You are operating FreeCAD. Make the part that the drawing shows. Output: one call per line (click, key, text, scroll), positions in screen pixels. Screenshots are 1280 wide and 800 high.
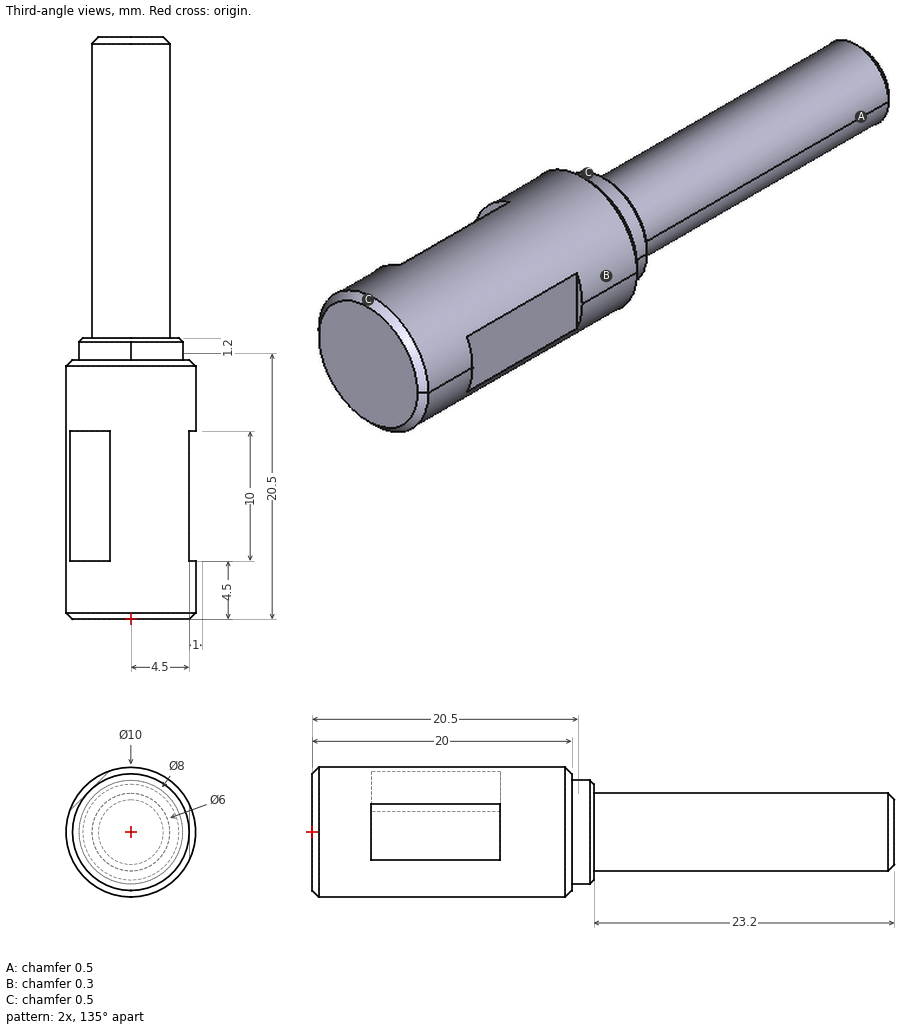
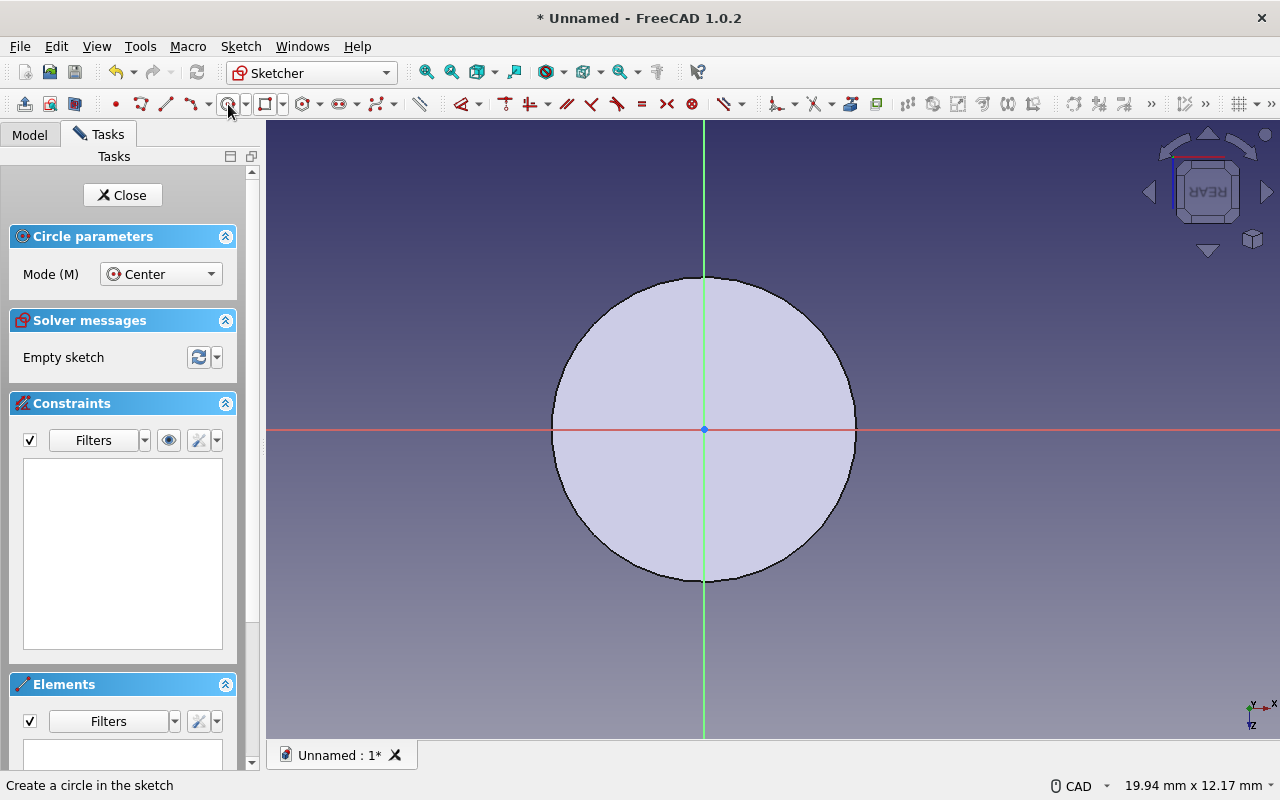
click(704, 429)
move(848, 286)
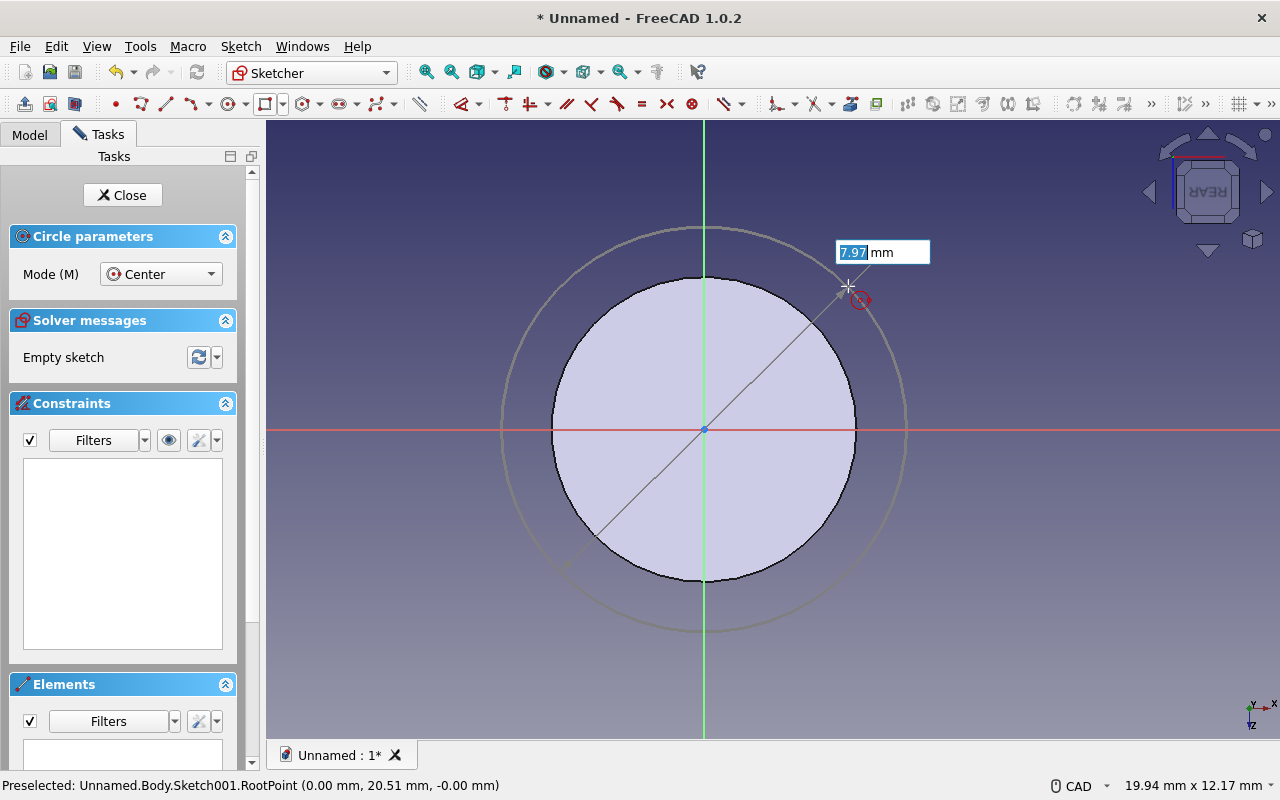
text(8)
key(Return)
key(Escape)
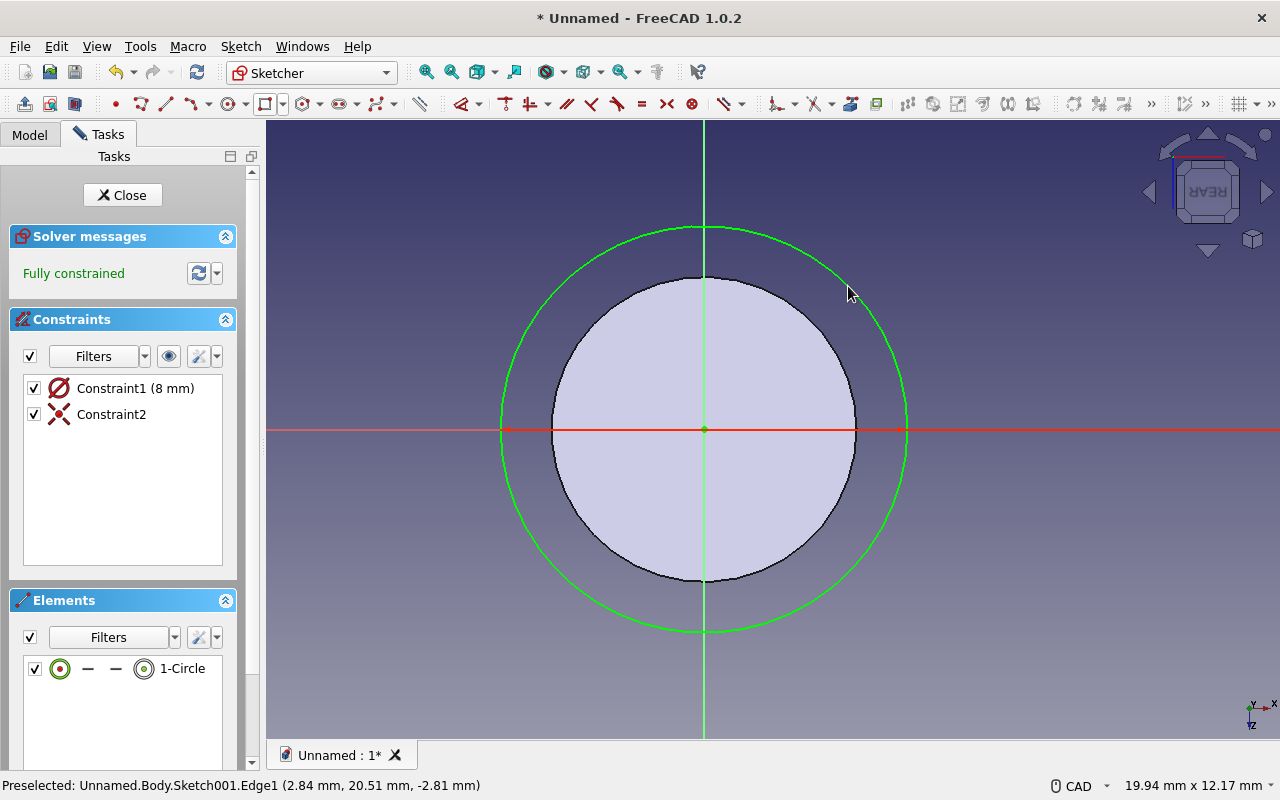
click(123, 195)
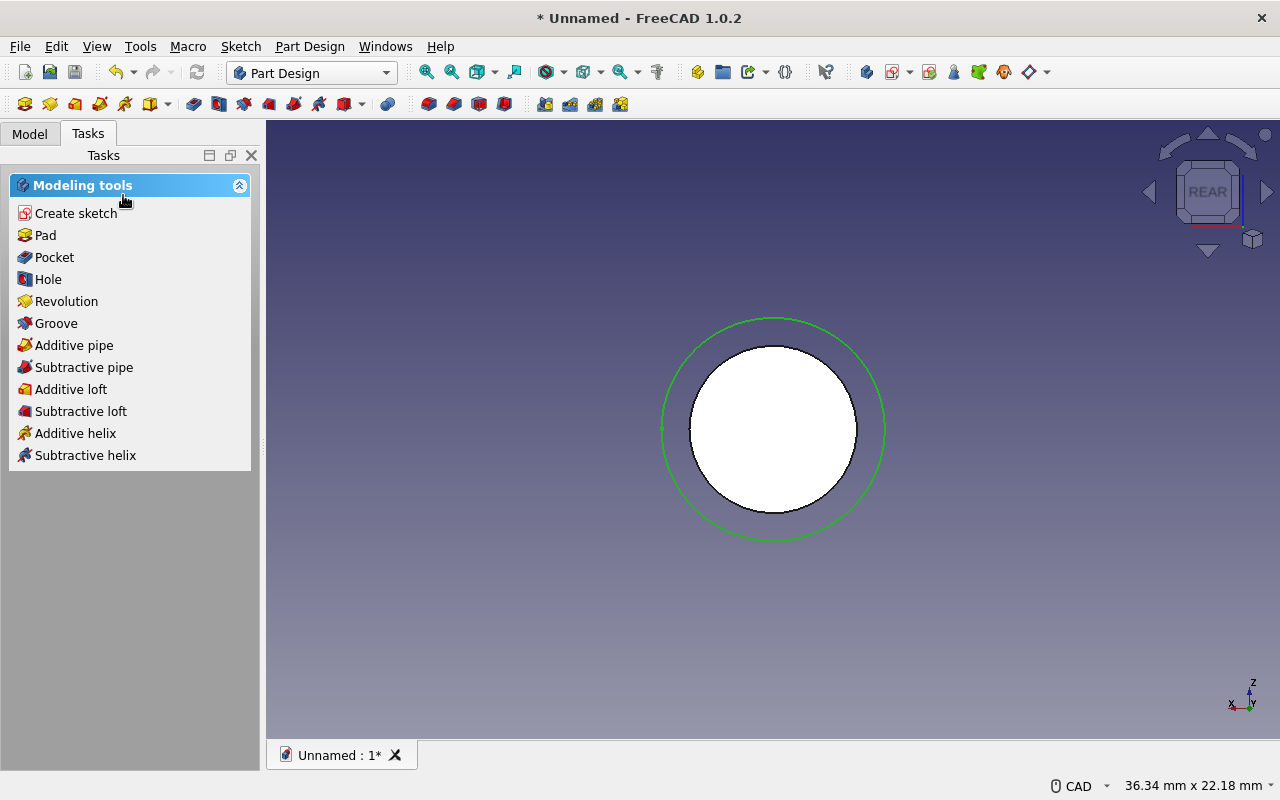
click(25, 104)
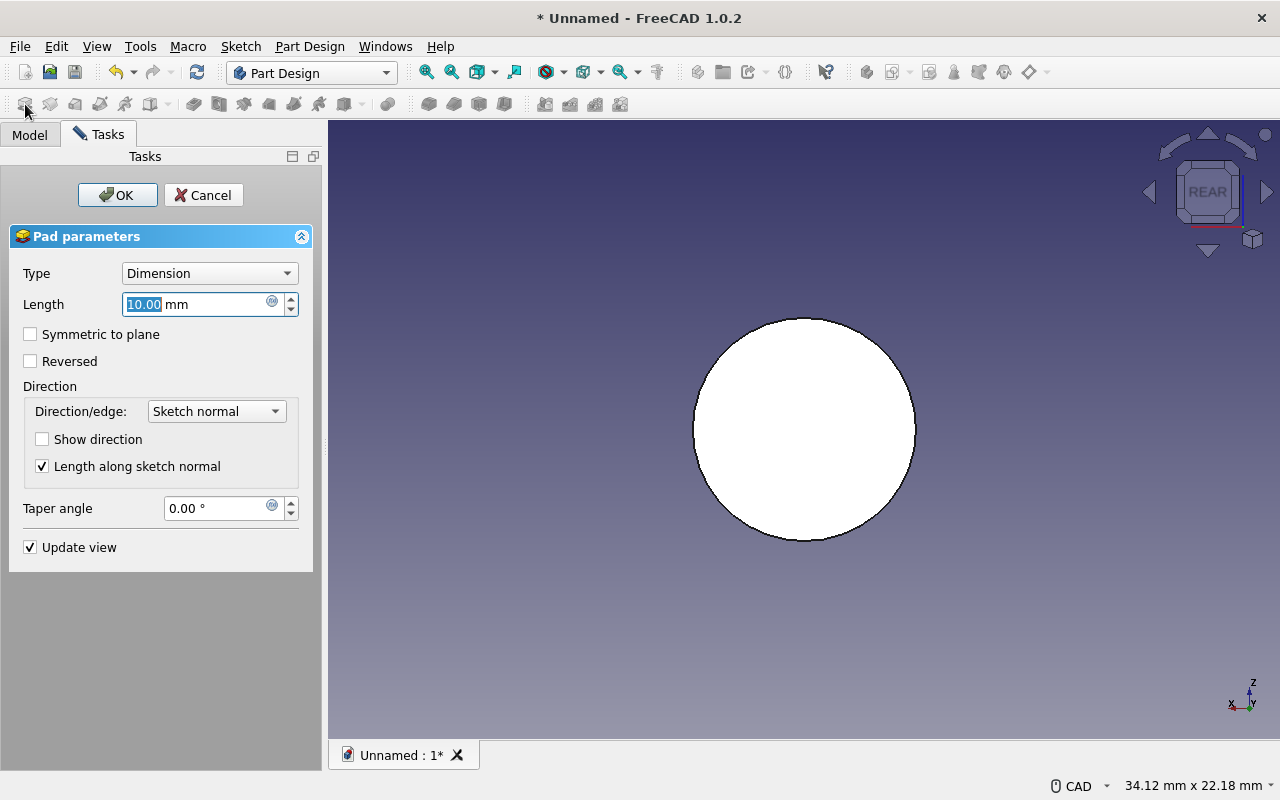
text(1.2)
key(Tab)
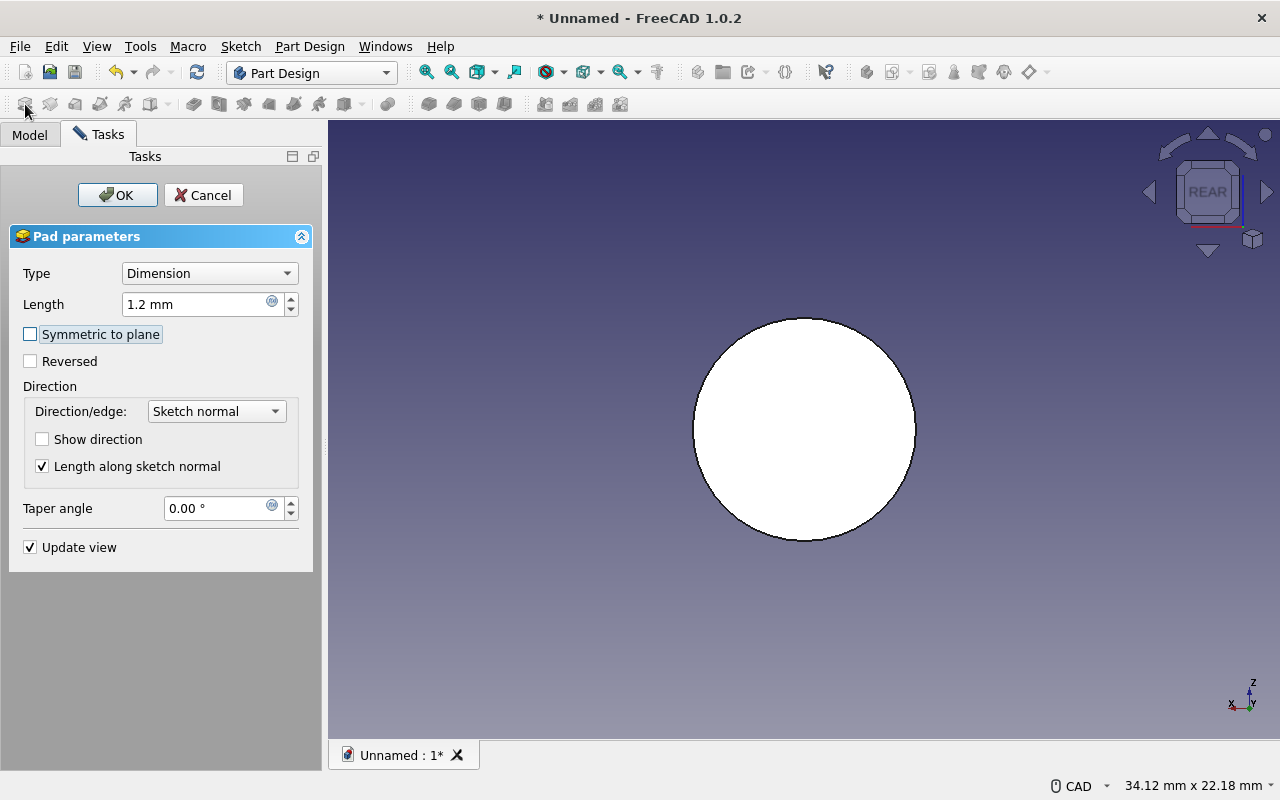
click(118, 195)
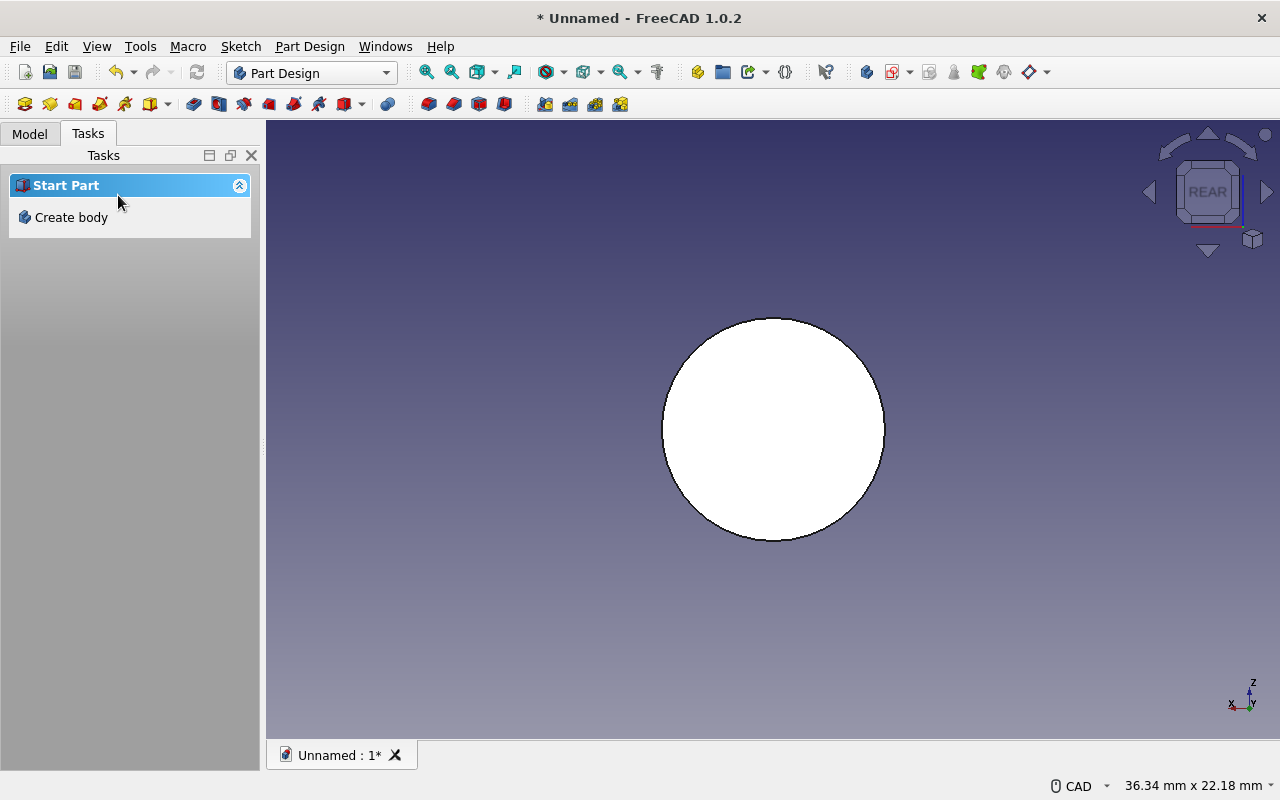
click(427, 72)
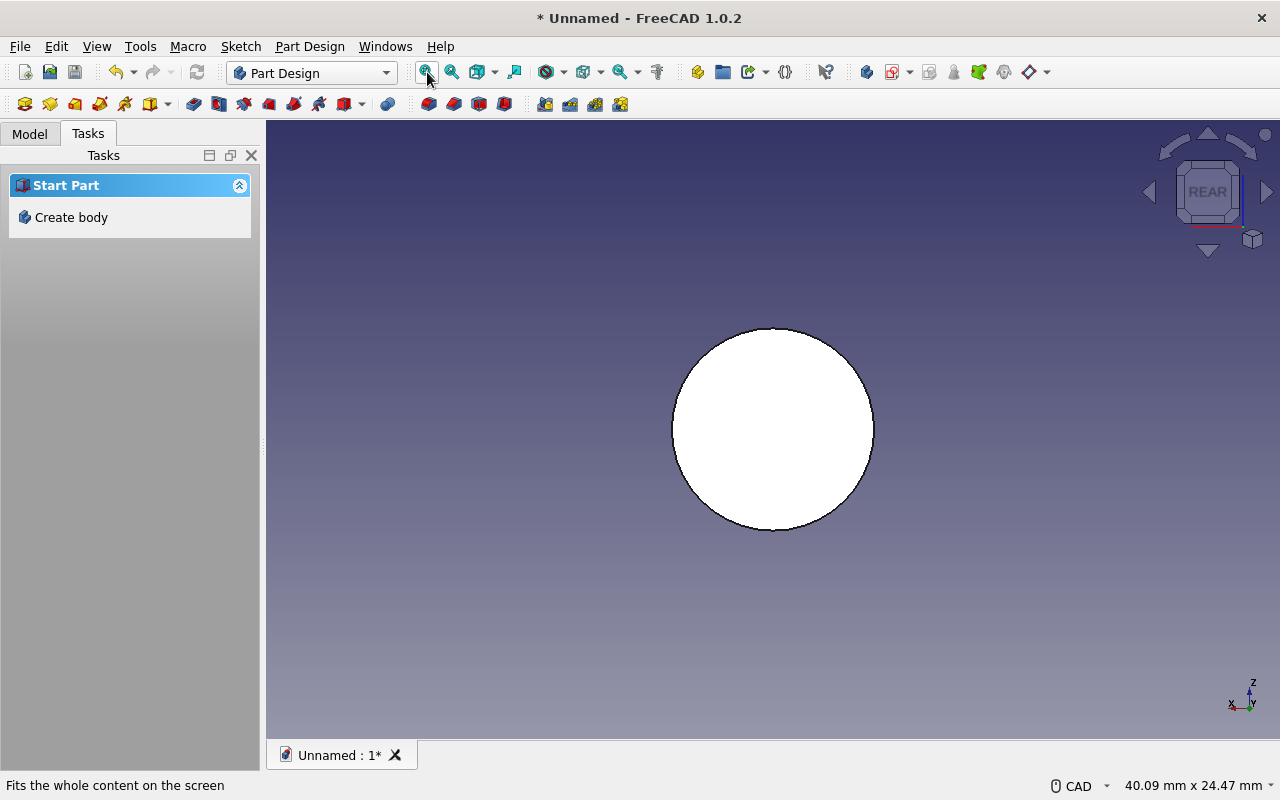
click(773, 428)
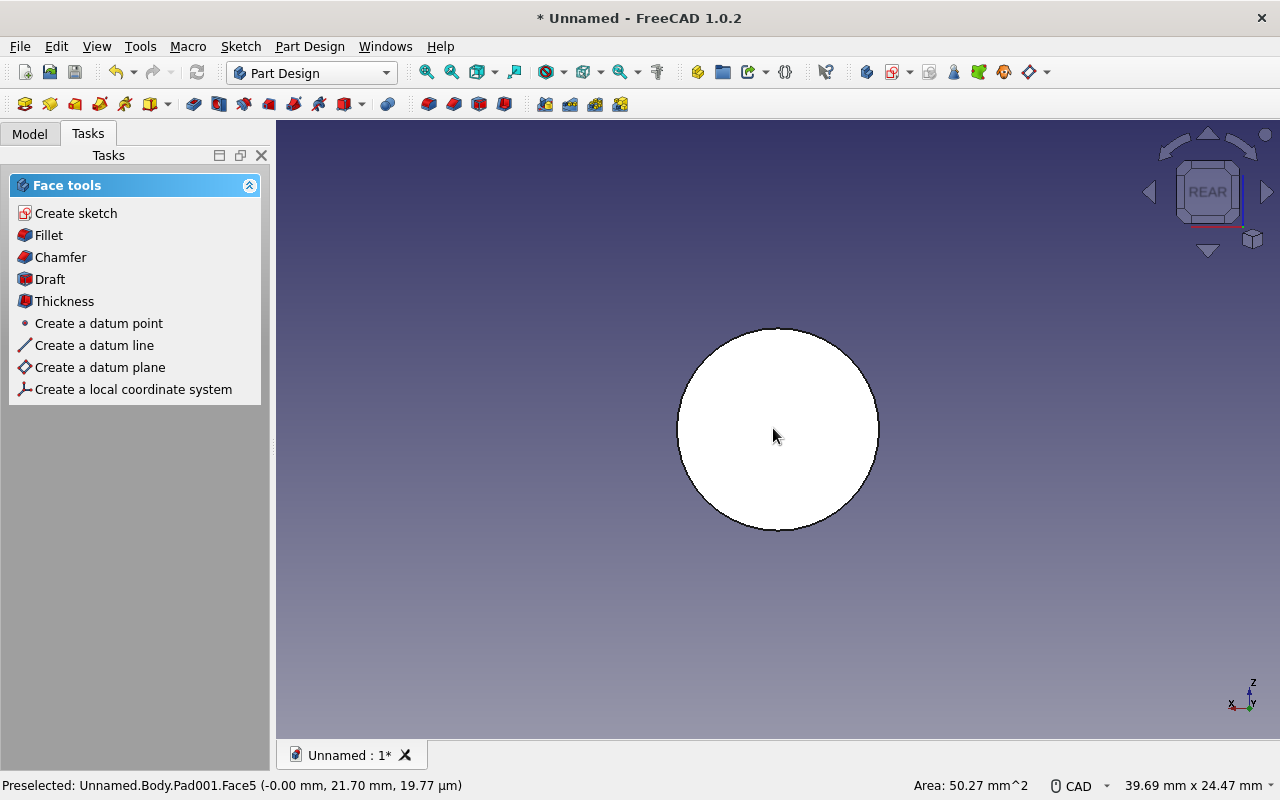
click(892, 72)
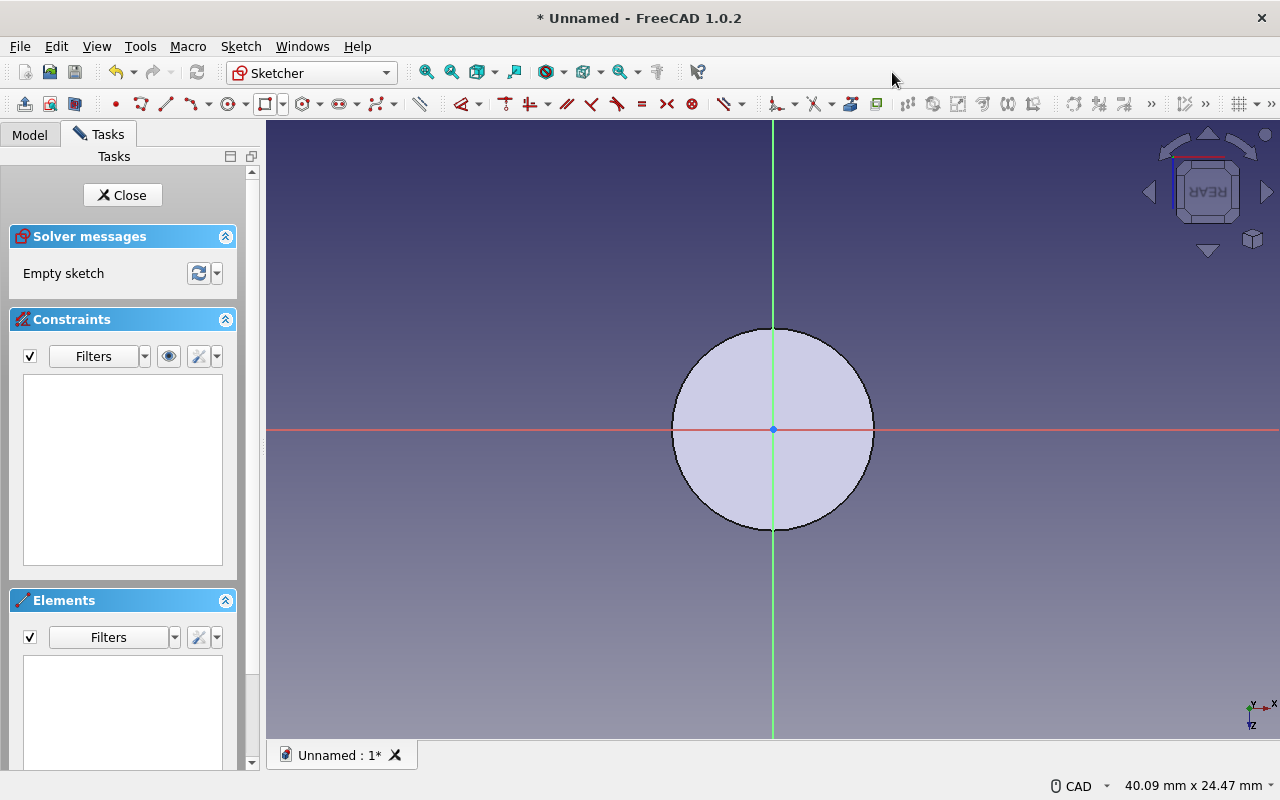
scroll(813, 429, up, 5)